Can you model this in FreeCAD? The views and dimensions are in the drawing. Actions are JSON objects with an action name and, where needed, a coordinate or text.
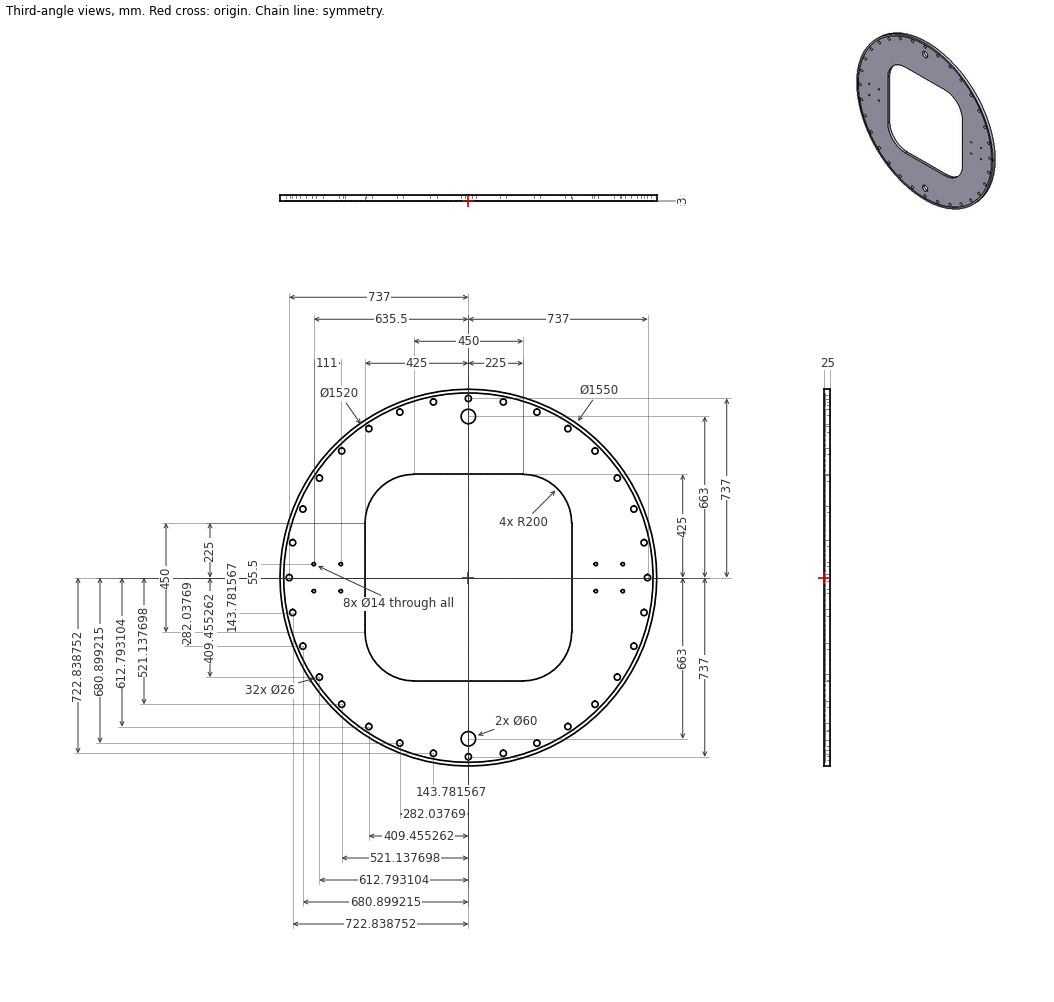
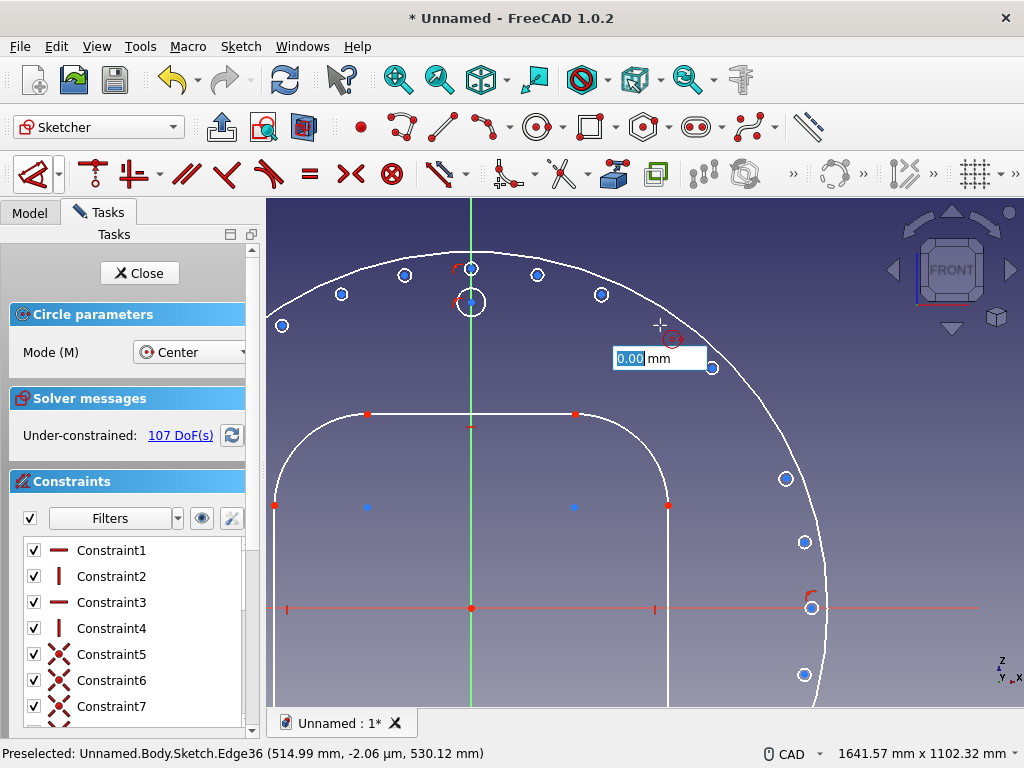
{"action": "scroll", "coordinate": [656, 321], "scroll_direction": "up", "scroll_amount": 5}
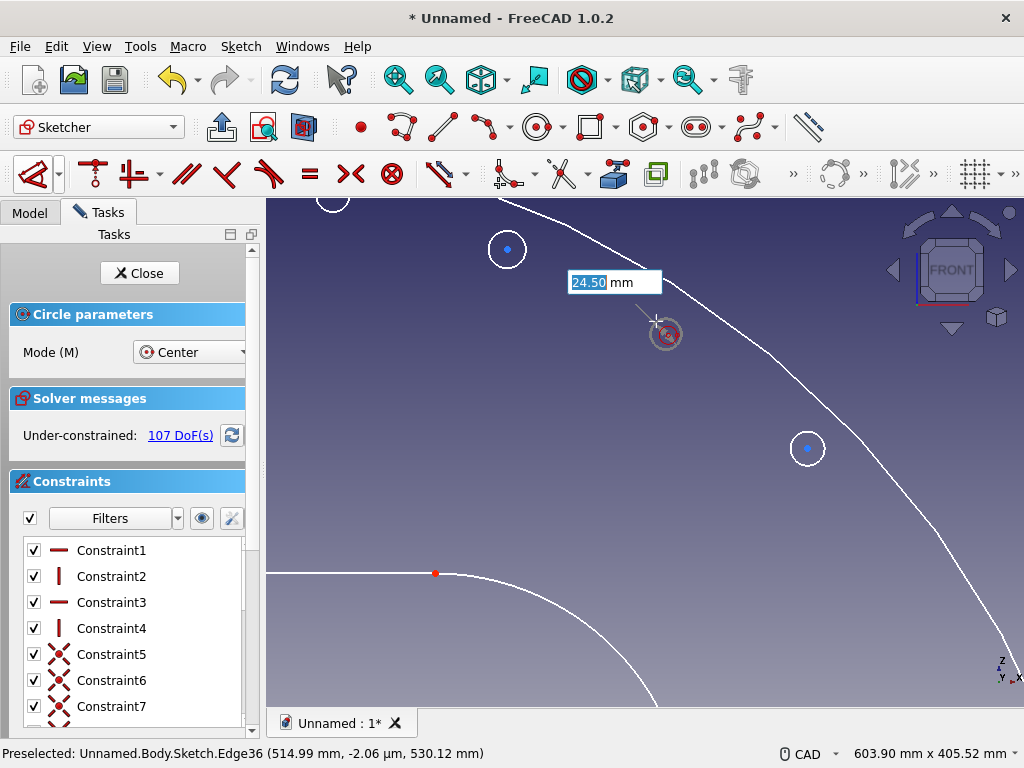
{"action": "left_click", "coordinate": [655, 320]}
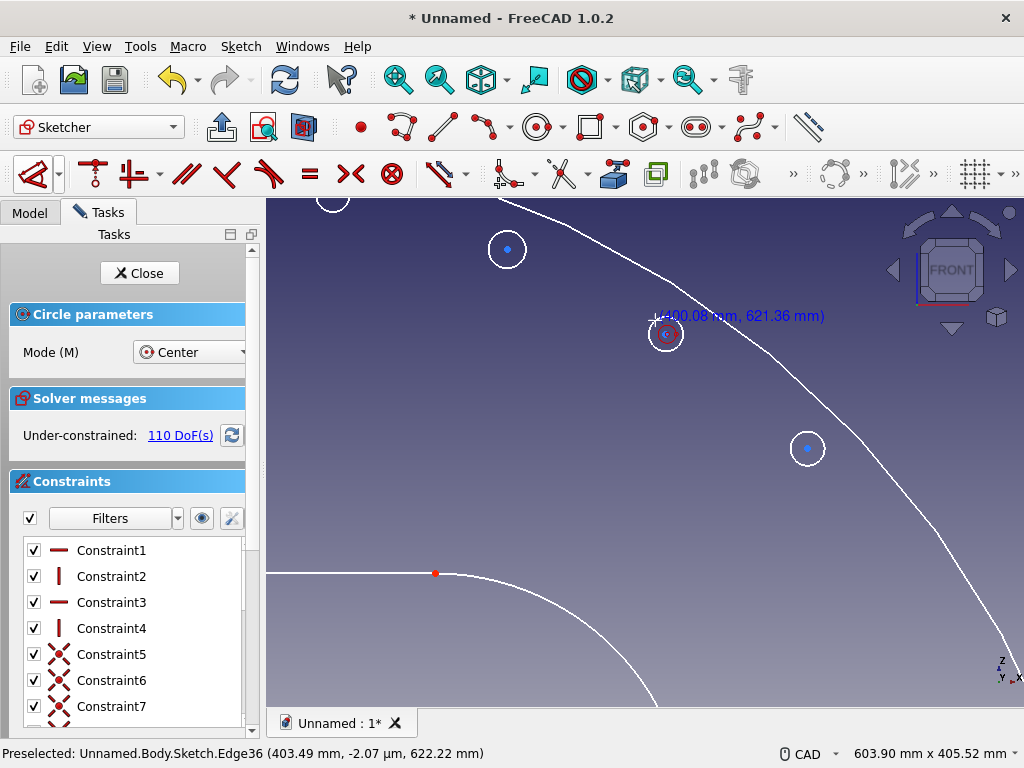
{"action": "scroll", "coordinate": [660, 324], "scroll_direction": "down", "scroll_amount": 9}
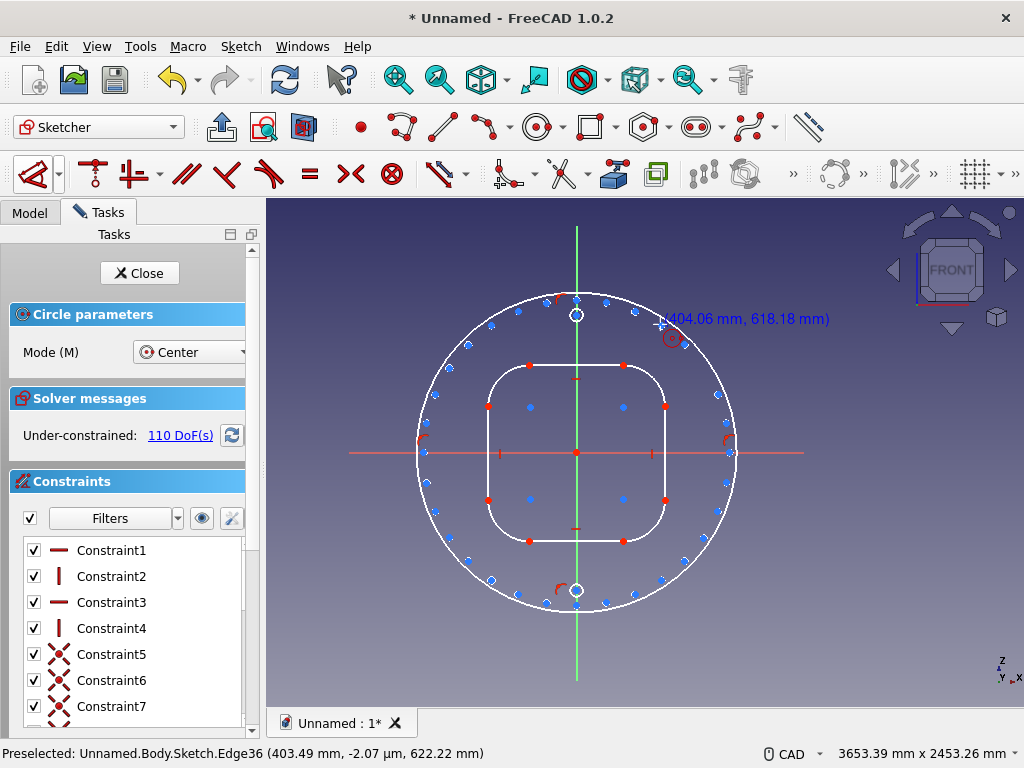
{"action": "scroll", "coordinate": [704, 368], "scroll_direction": "up", "scroll_amount": 11}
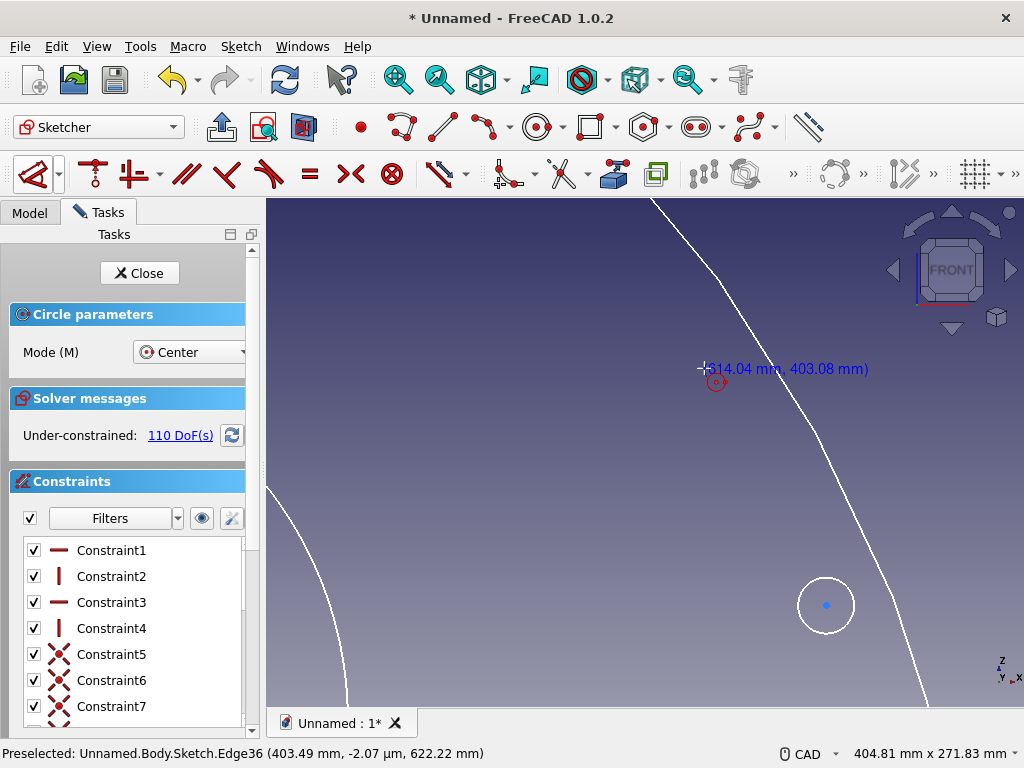
{"action": "scroll", "coordinate": [704, 368], "scroll_direction": "down", "scroll_amount": 11}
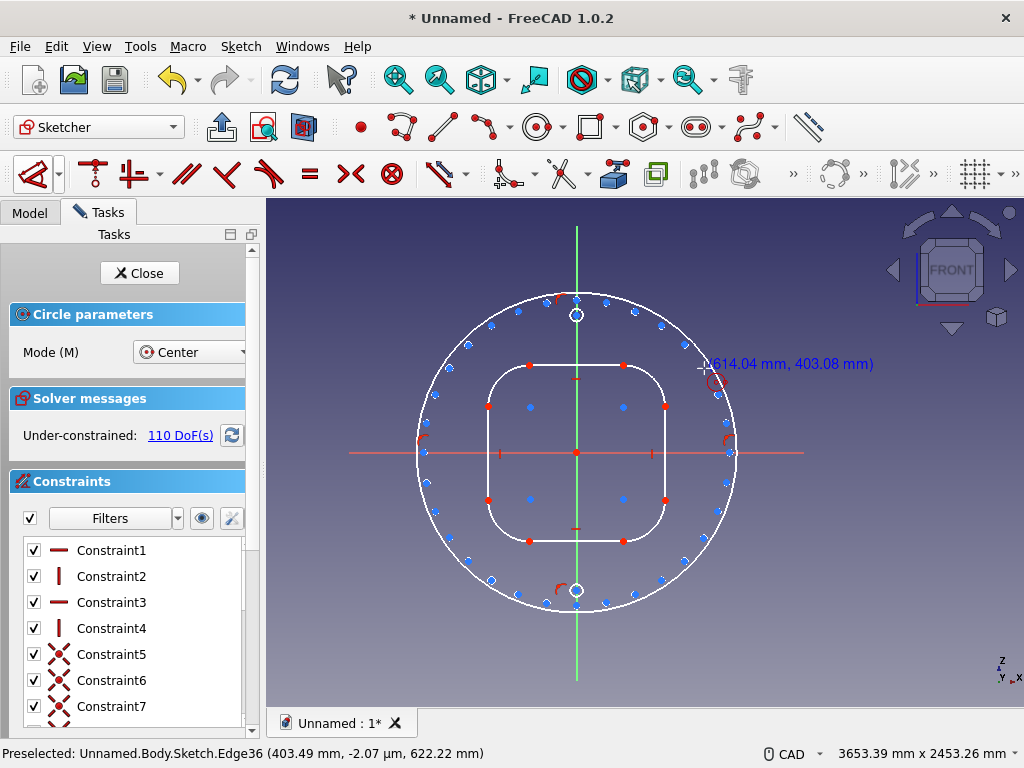
{"action": "scroll", "coordinate": [704, 368], "scroll_direction": "up", "scroll_amount": 4}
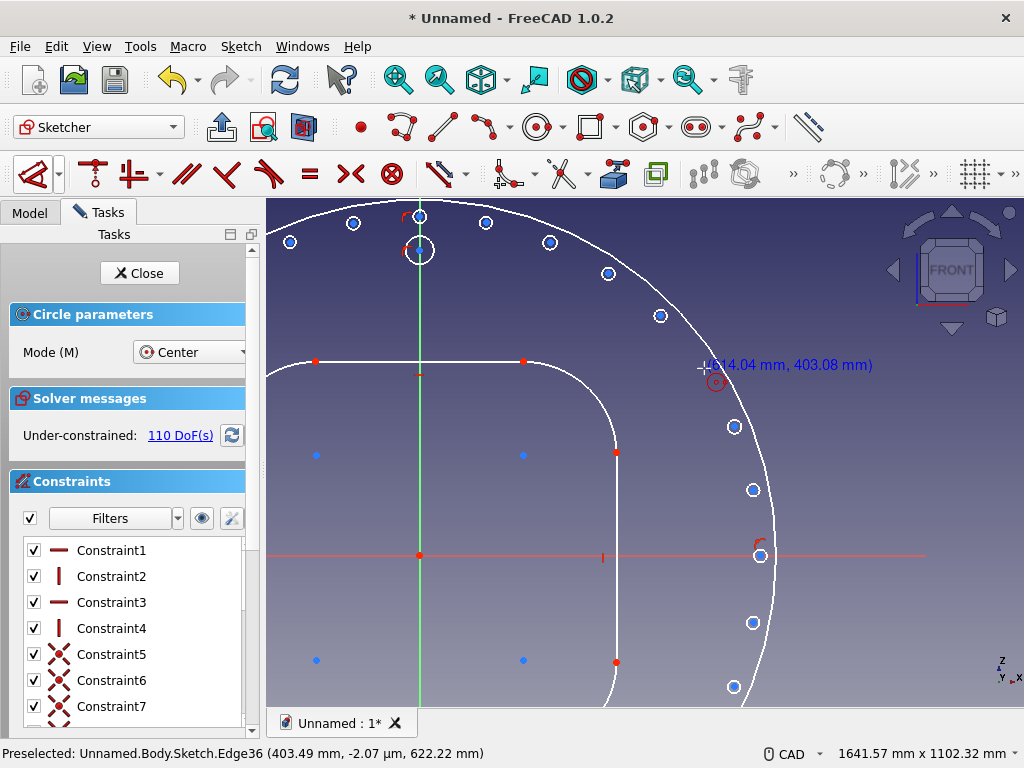
{"action": "left_click", "coordinate": [703, 367]}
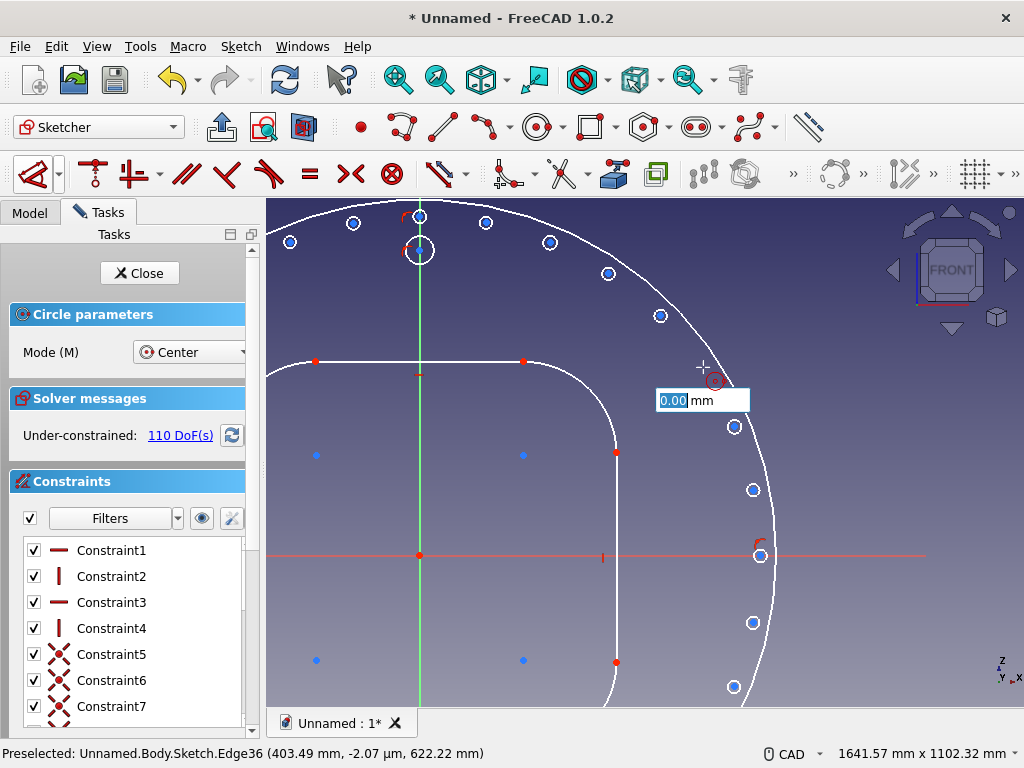
{"action": "scroll", "coordinate": [698, 363], "scroll_direction": "up", "scroll_amount": 5}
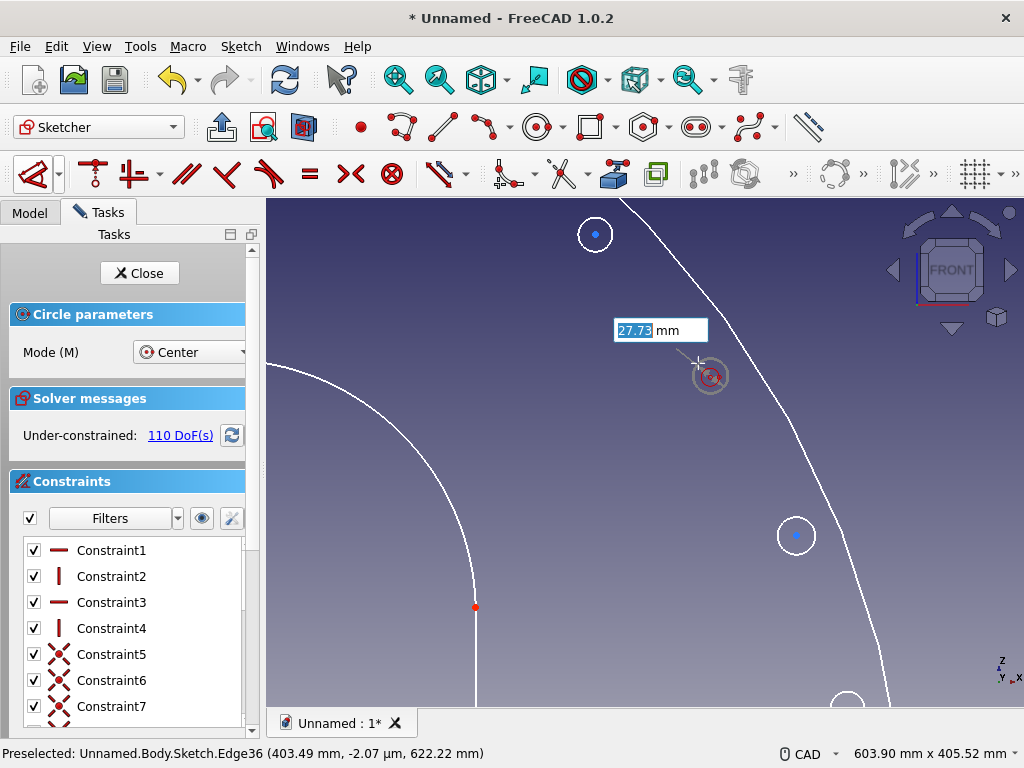
{"action": "left_click", "coordinate": [698, 361]}
{"action": "key", "text": "Escape"}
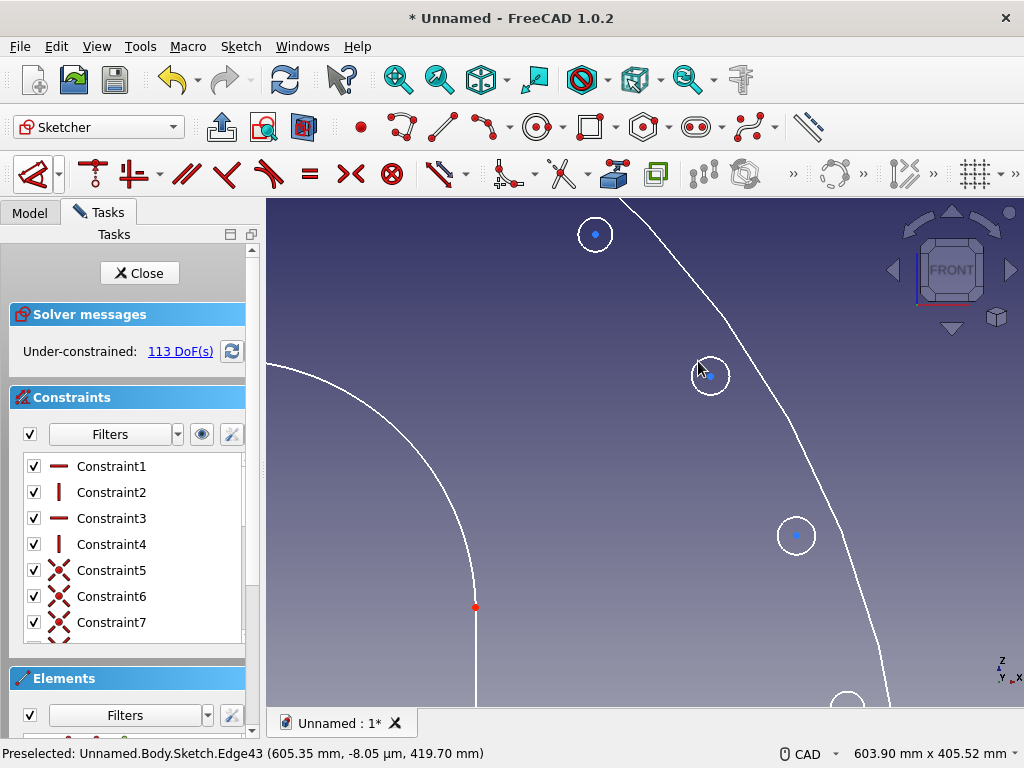
{"action": "scroll", "coordinate": [702, 366], "scroll_direction": "down", "scroll_amount": 9}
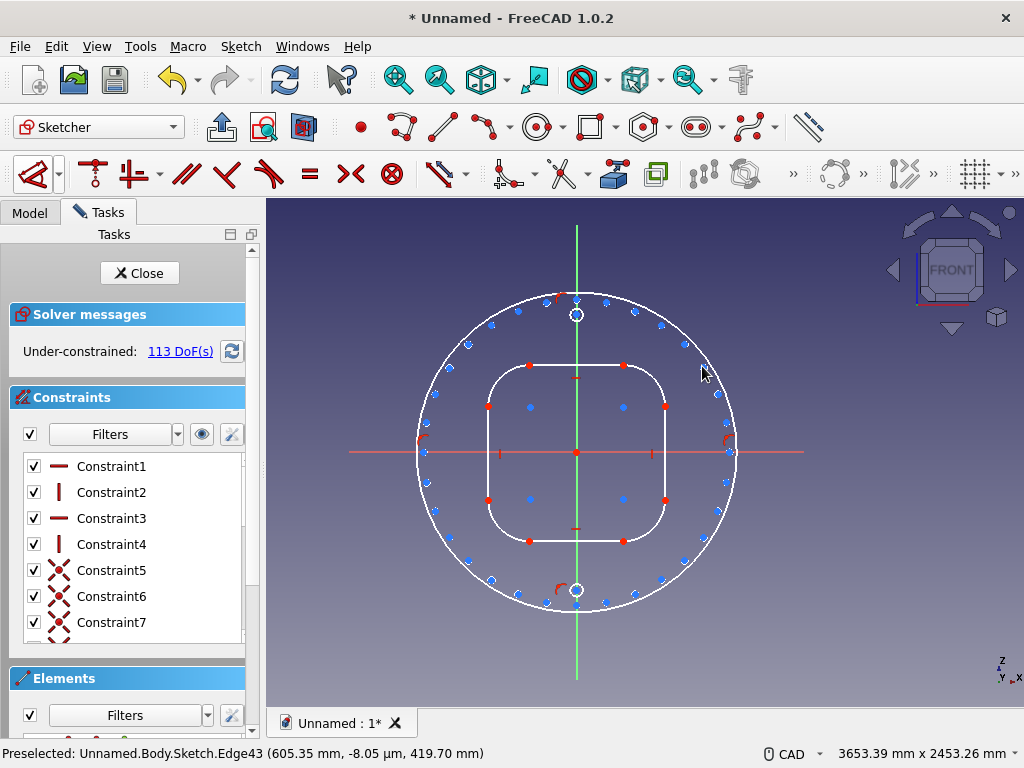
{"action": "left_click", "coordinate": [511, 370]}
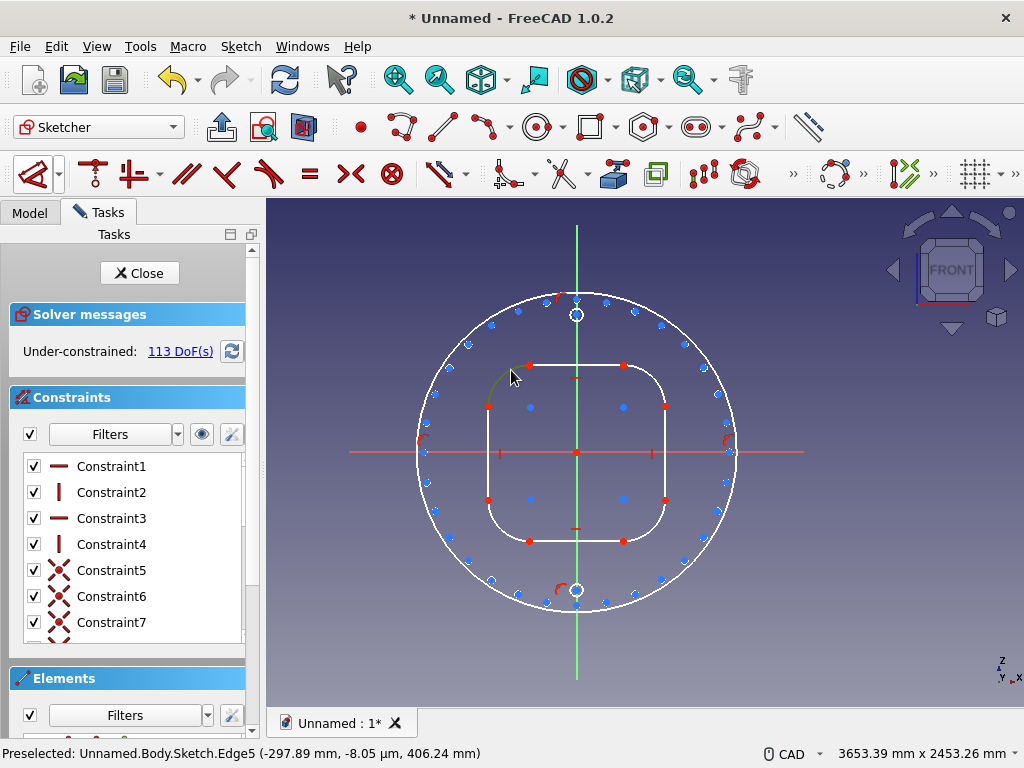
{"action": "left_click", "coordinate": [493, 519]}